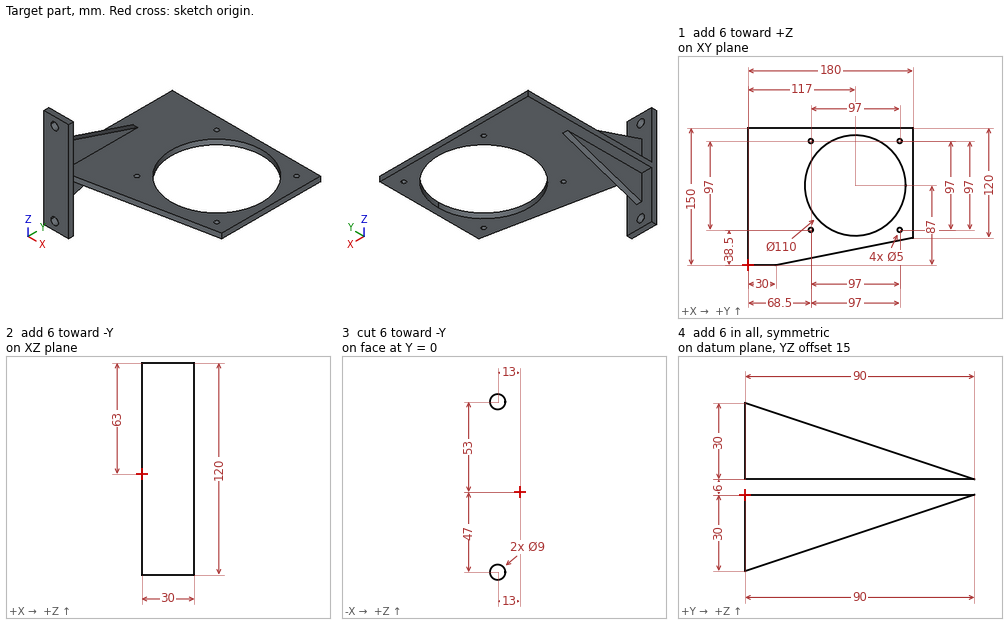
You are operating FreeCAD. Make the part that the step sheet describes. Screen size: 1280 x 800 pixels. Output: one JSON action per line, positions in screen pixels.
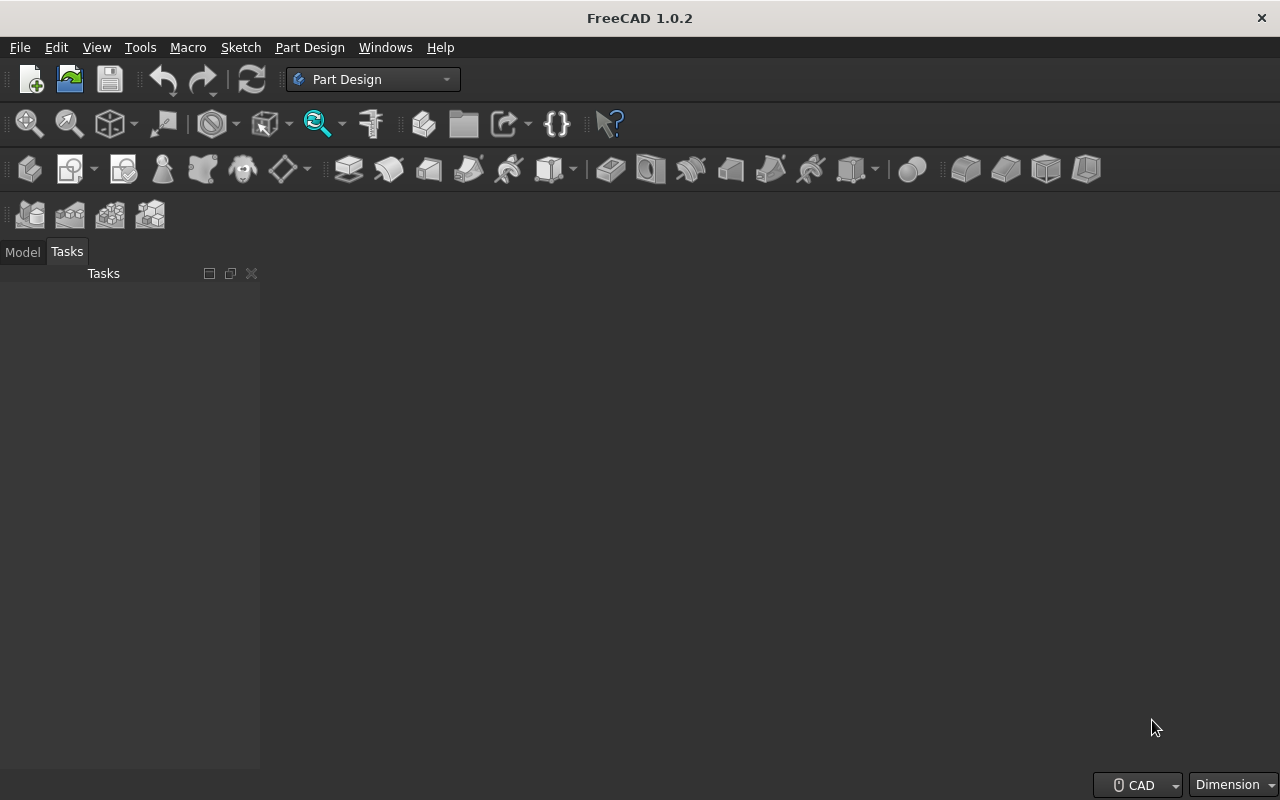
{"action": "left_click", "coordinate": [30, 80]}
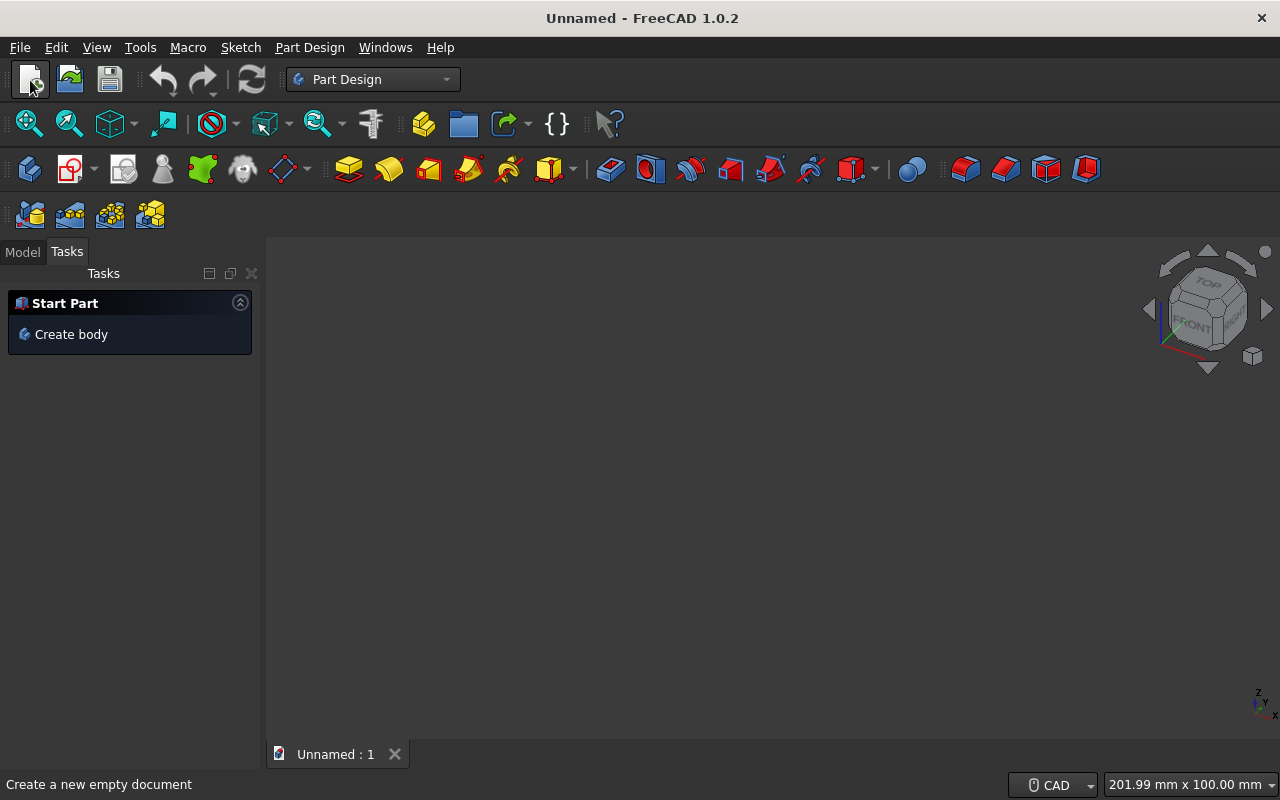
{"action": "left_click", "coordinate": [70, 170]}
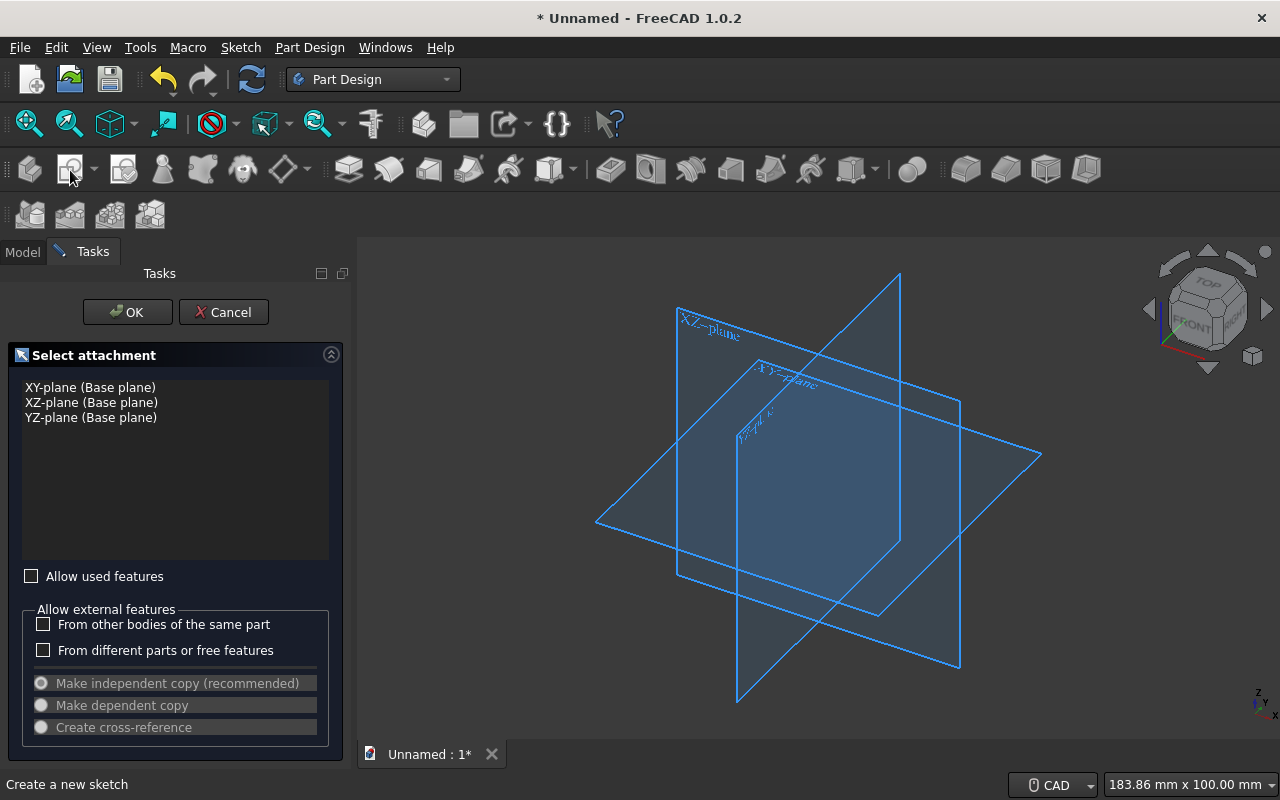
{"action": "left_click", "coordinate": [82, 388]}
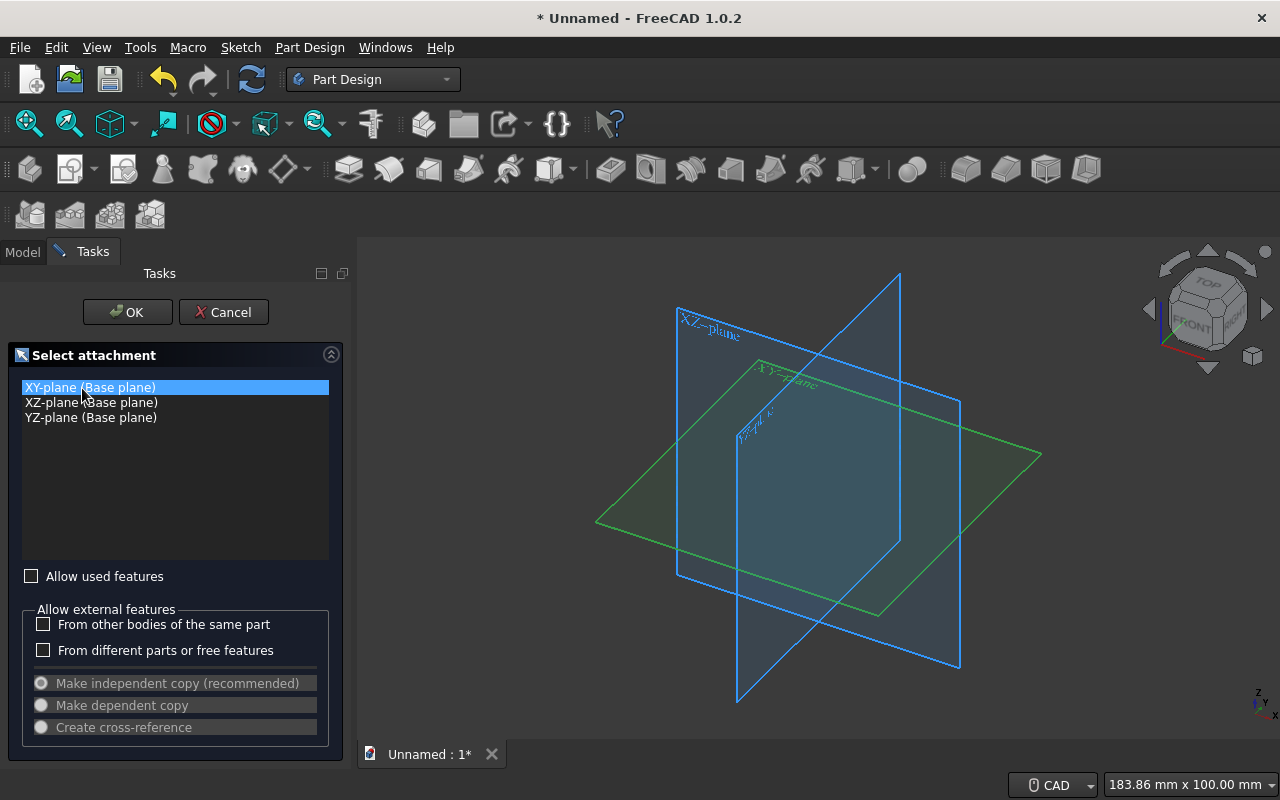
{"action": "left_click", "coordinate": [128, 312]}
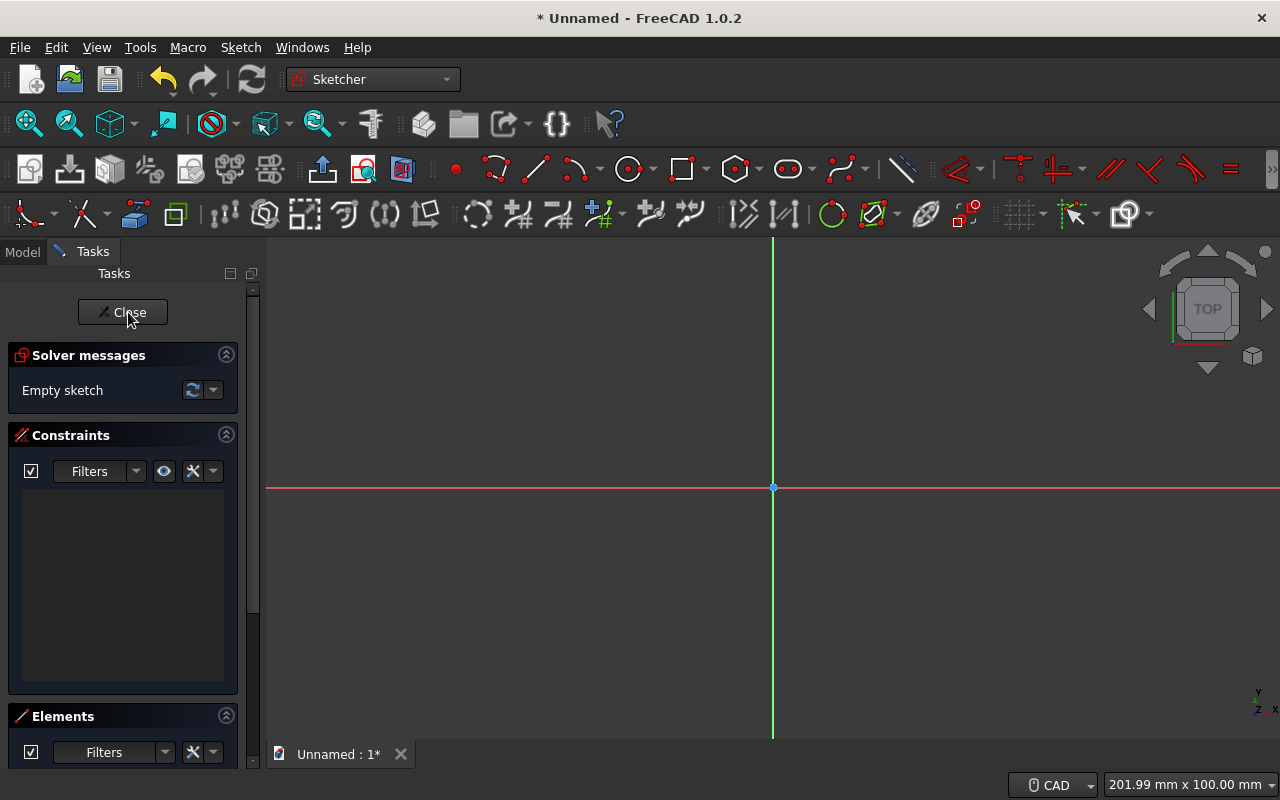
{"action": "scroll", "coordinate": [402, 707], "scroll_direction": "down", "scroll_amount": 5}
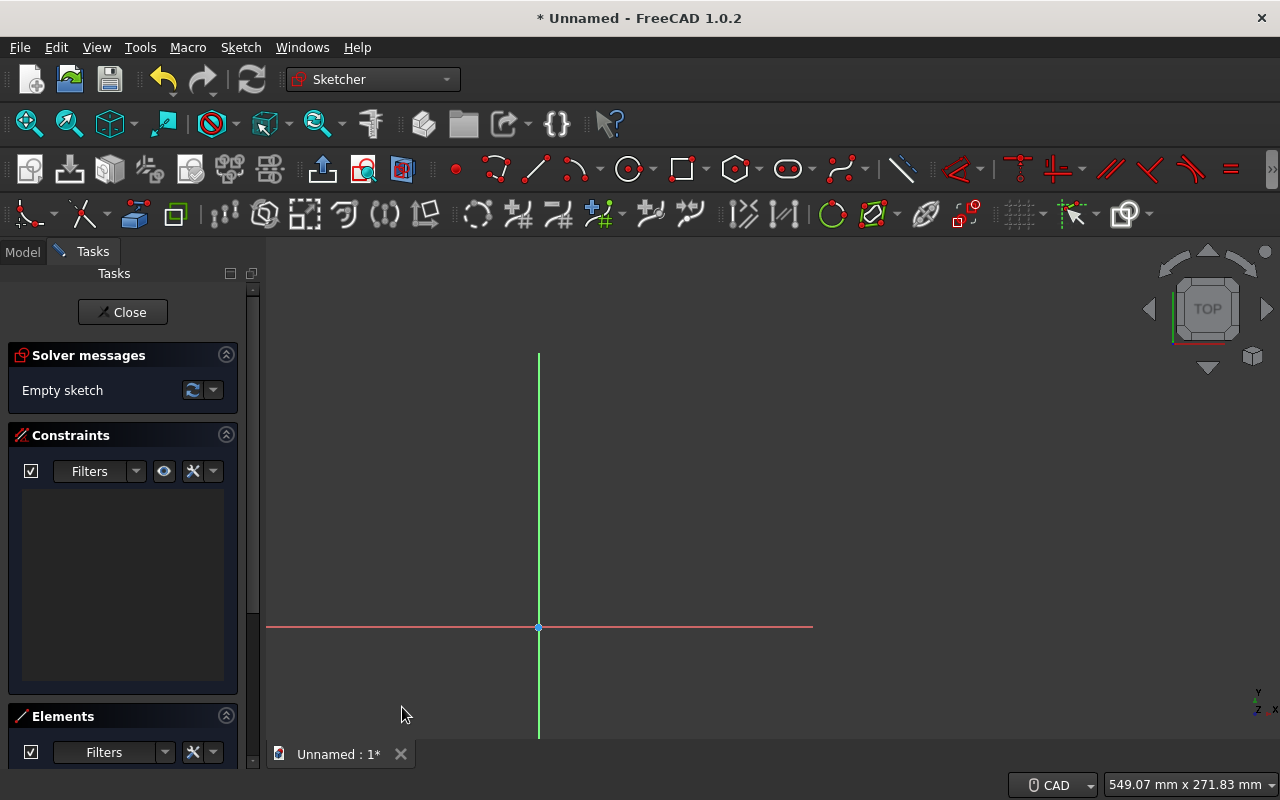
{"action": "key", "text": "g m"}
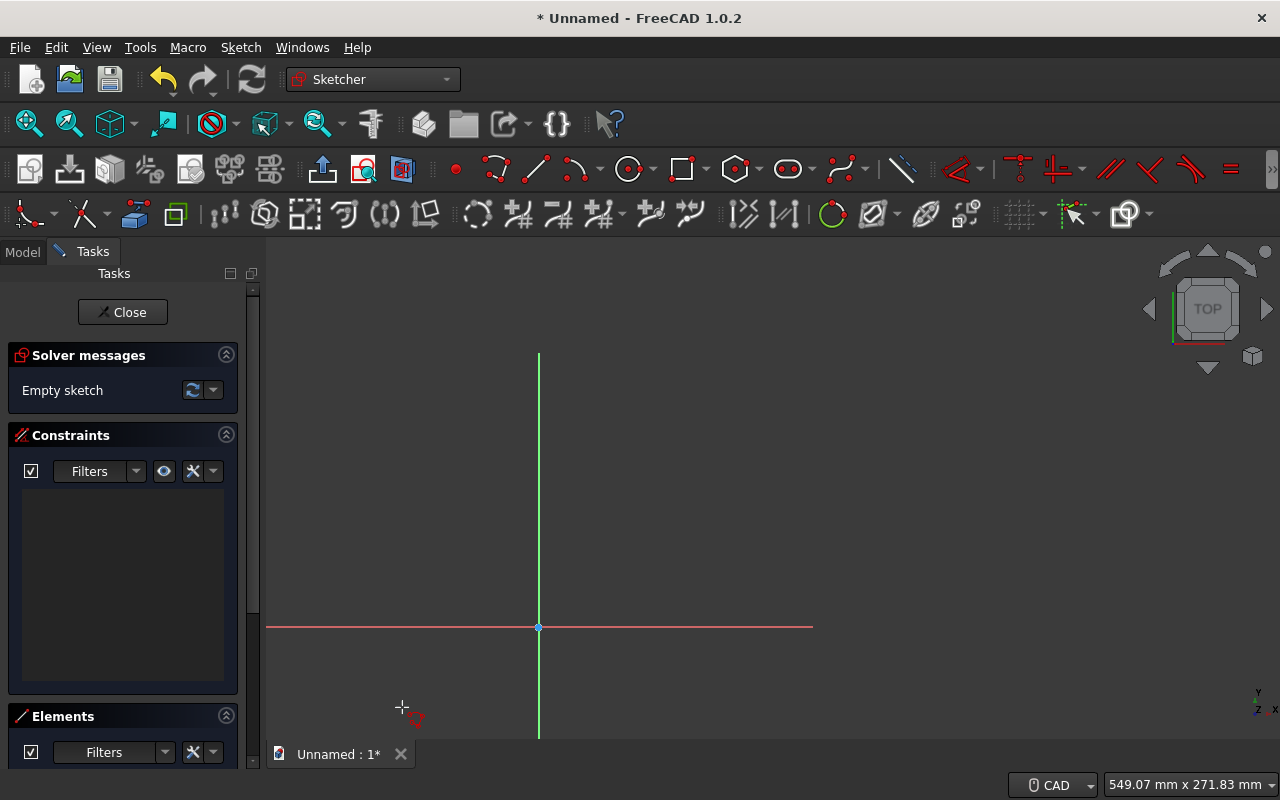
{"action": "left_click", "coordinate": [539, 627]}
{"action": "left_click", "coordinate": [594, 618]}
{"action": "left_click", "coordinate": [871, 572]}
{"action": "left_click", "coordinate": [871, 350]}
{"action": "left_click", "coordinate": [548, 350]}
{"action": "left_click", "coordinate": [539, 627]}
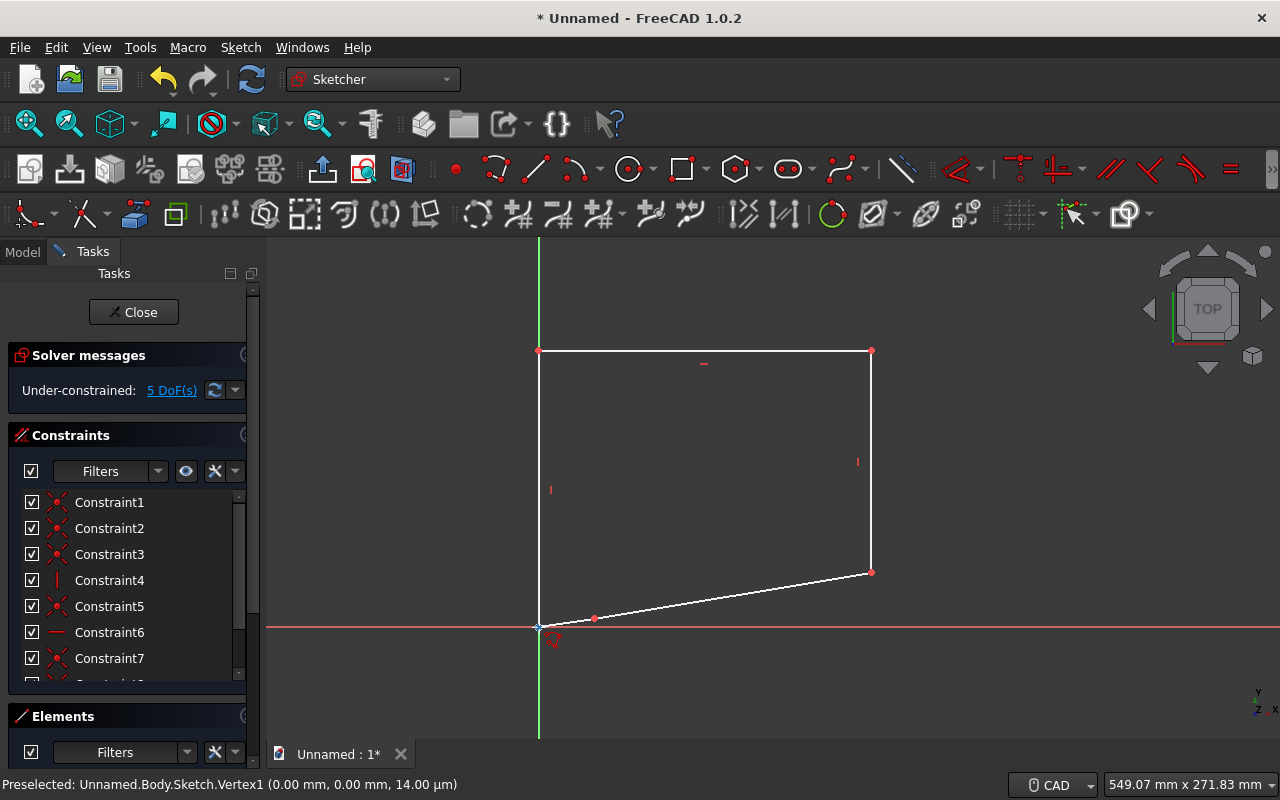
{"action": "key", "text": "g c"}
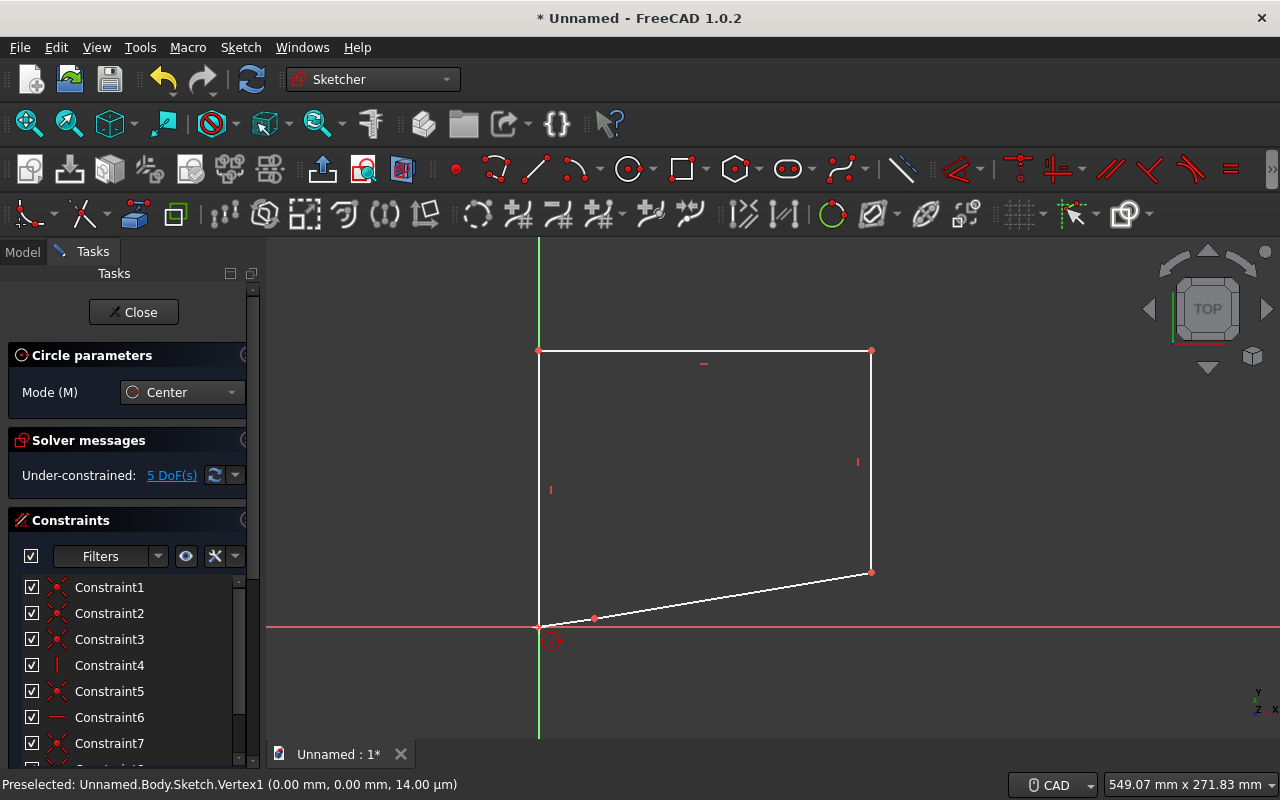
{"action": "scroll", "coordinate": [665, 556], "scroll_direction": "up", "scroll_amount": 8}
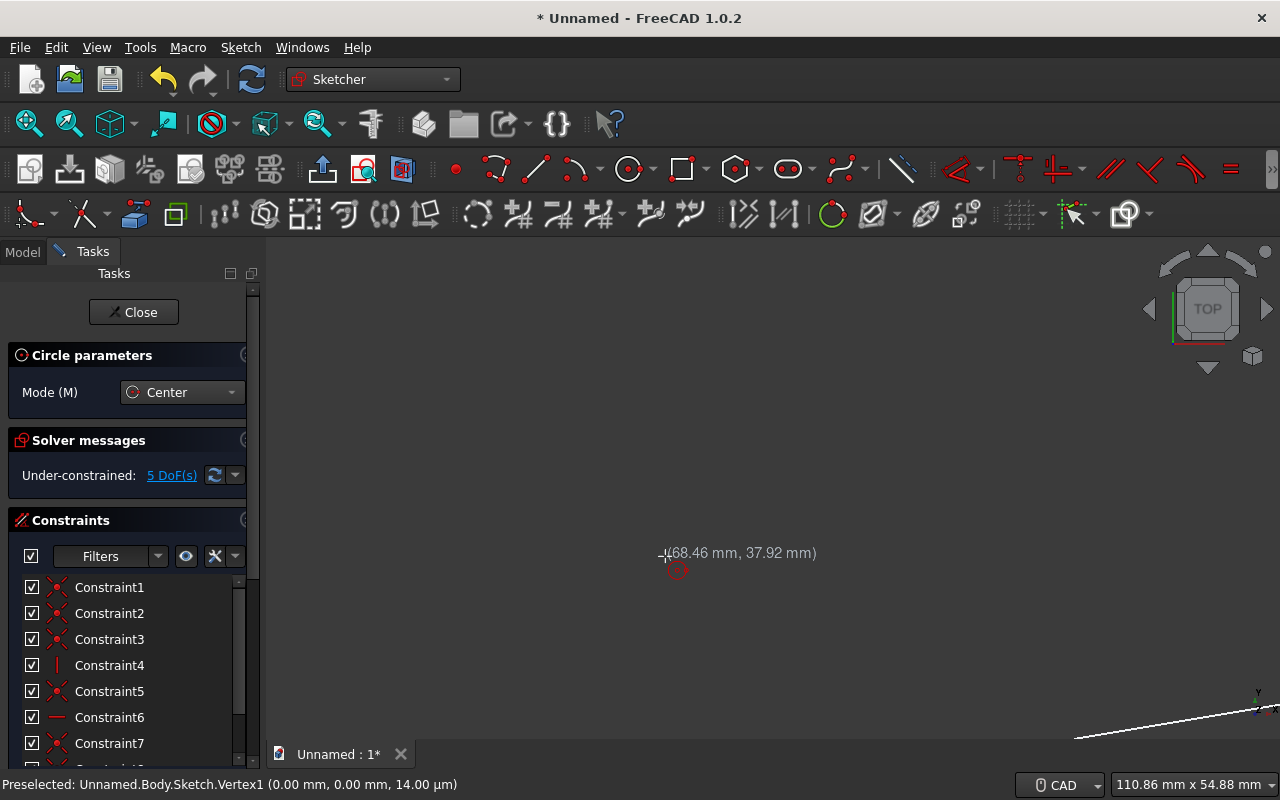
{"action": "scroll", "coordinate": [653, 576], "scroll_direction": "down", "scroll_amount": 7}